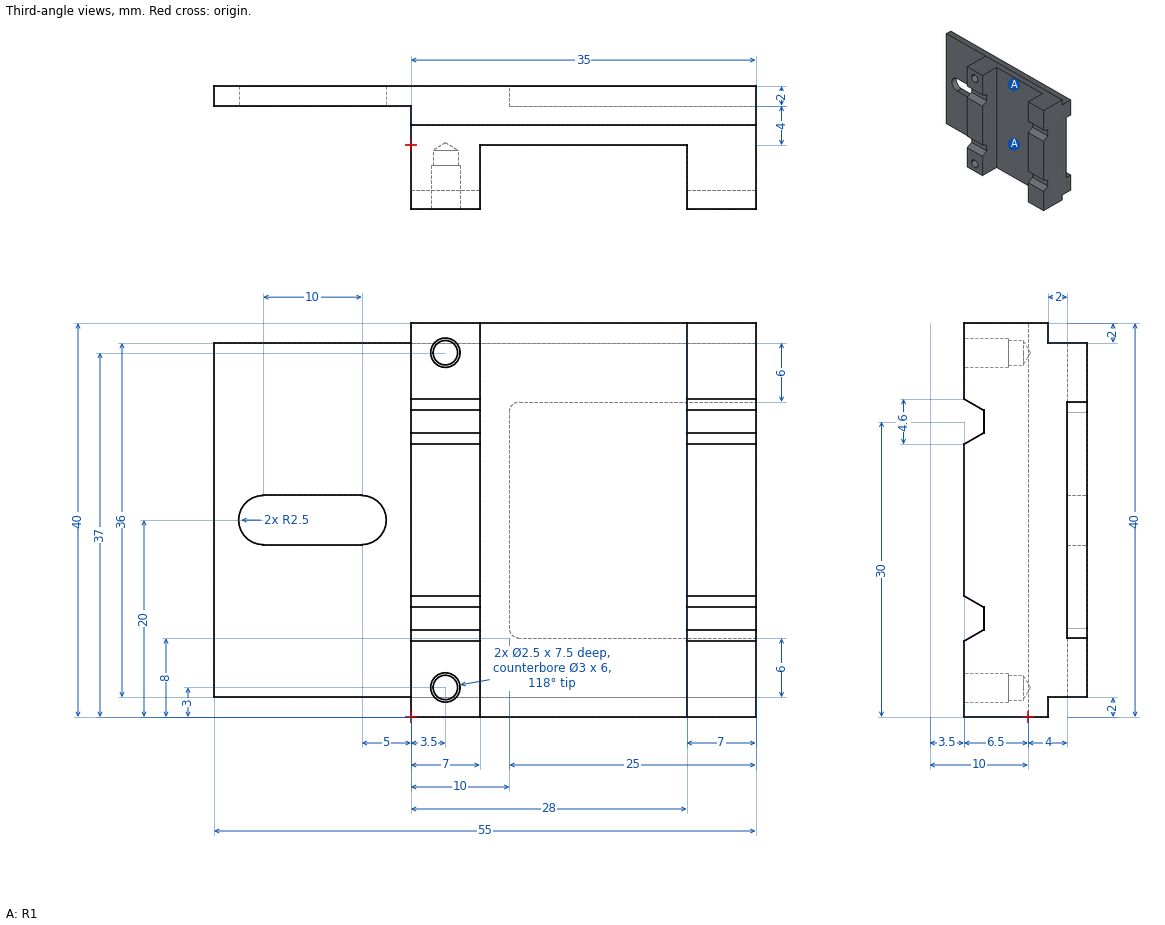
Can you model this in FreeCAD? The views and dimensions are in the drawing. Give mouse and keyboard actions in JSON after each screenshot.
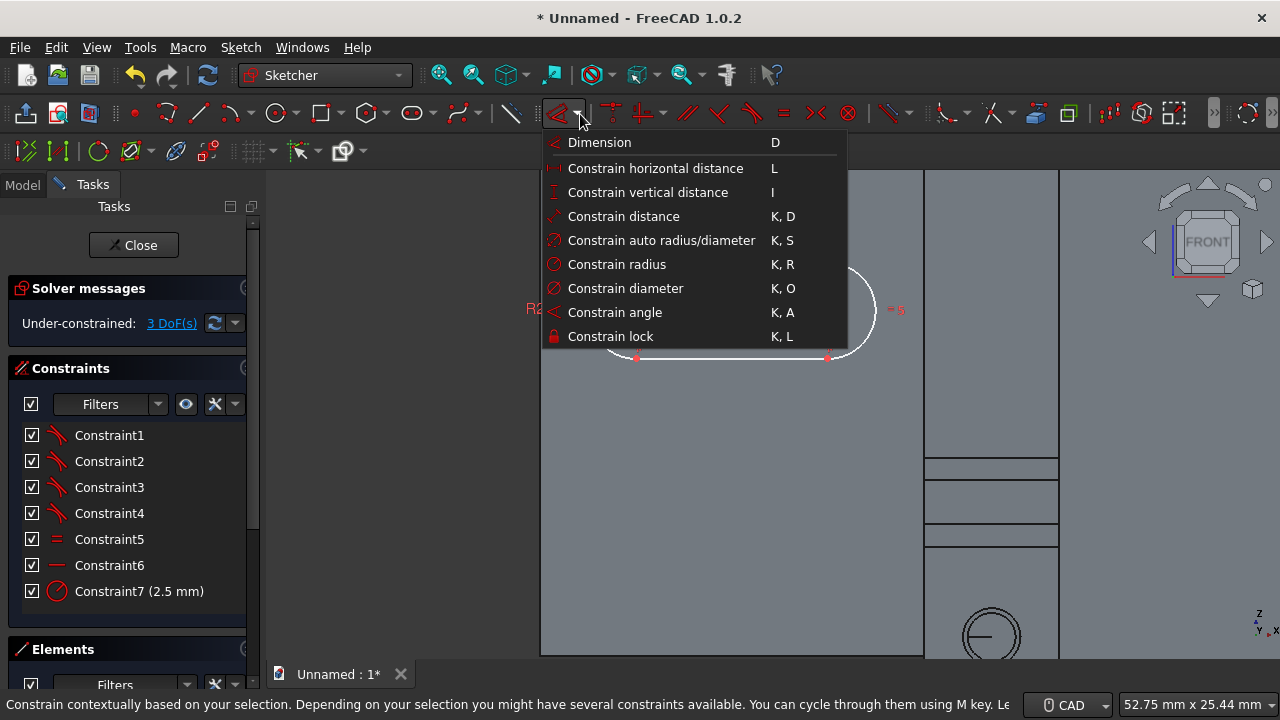
{"action": "left_click", "coordinate": [695, 168]}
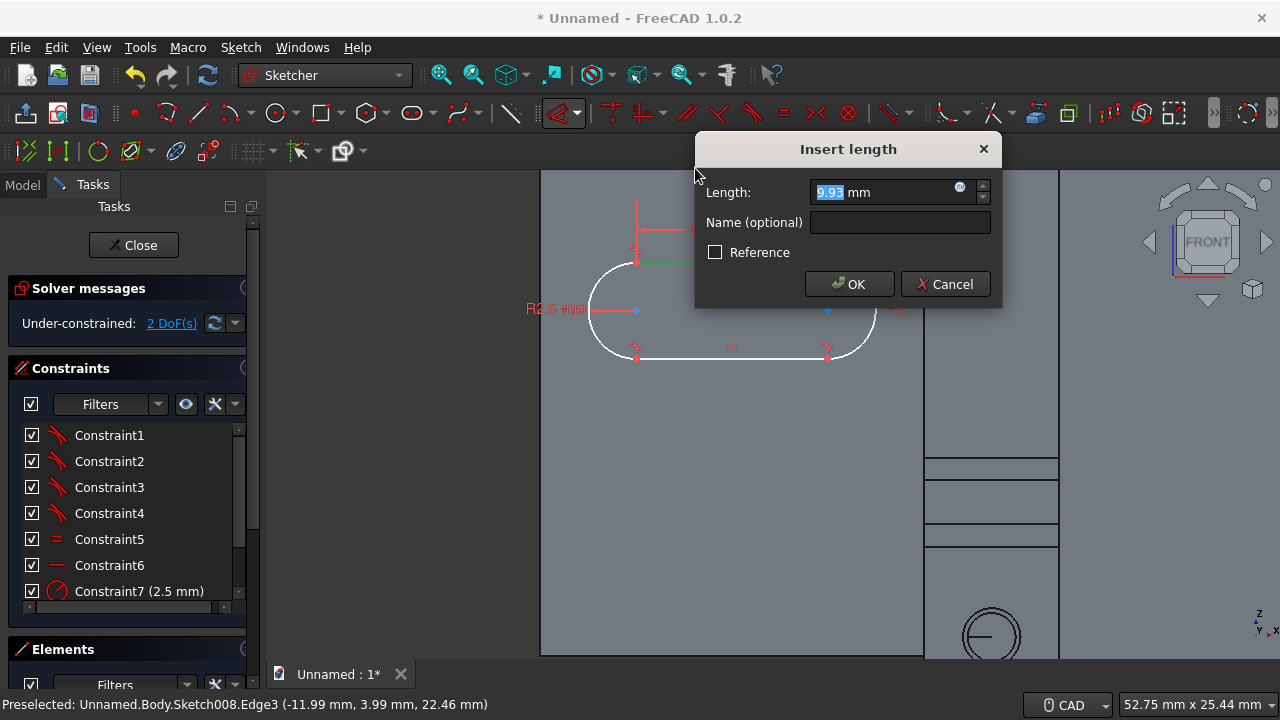
{"action": "type", "text": "10"}
{"action": "key", "text": "Return"}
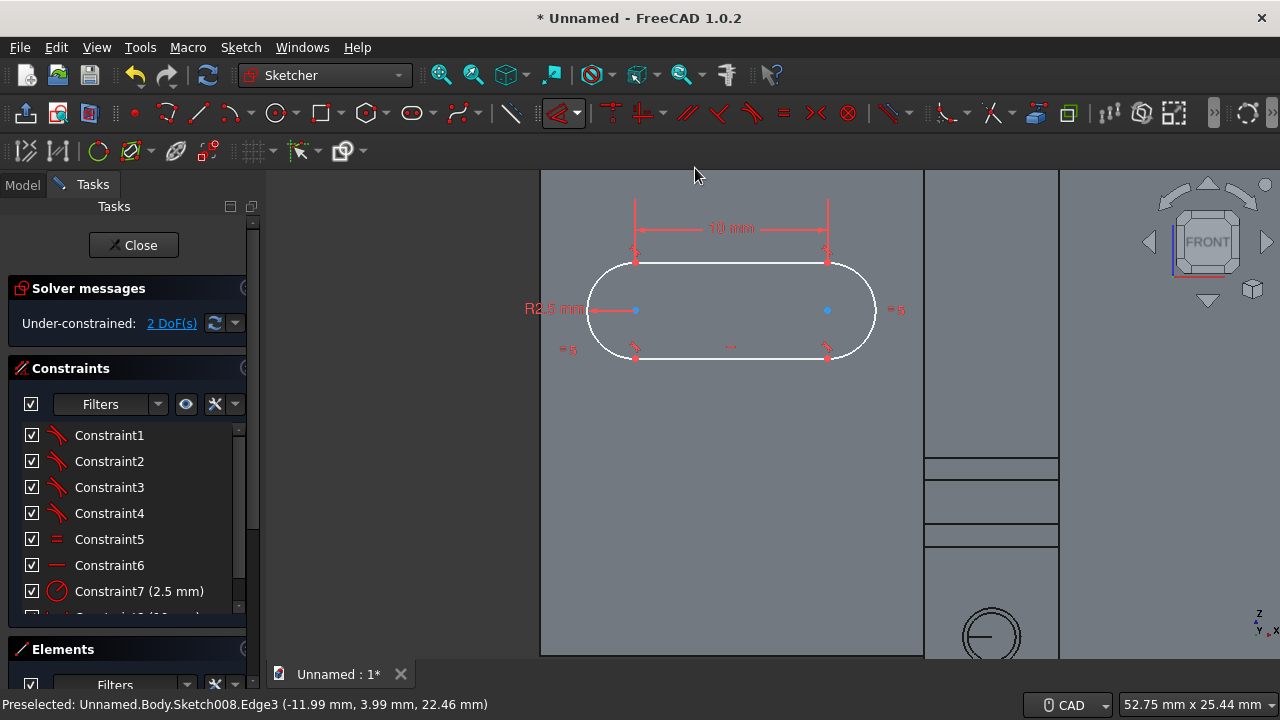
{"action": "left_click", "coordinate": [828, 359]}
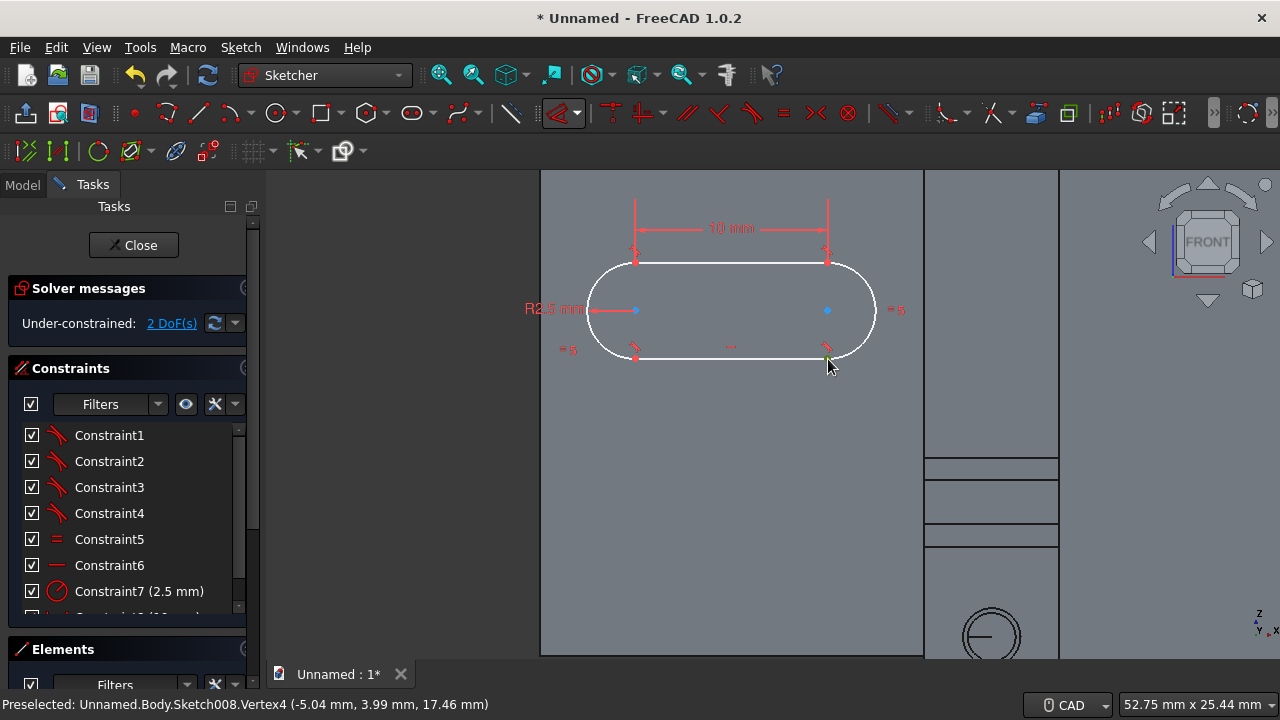
{"action": "key", "text": "l"}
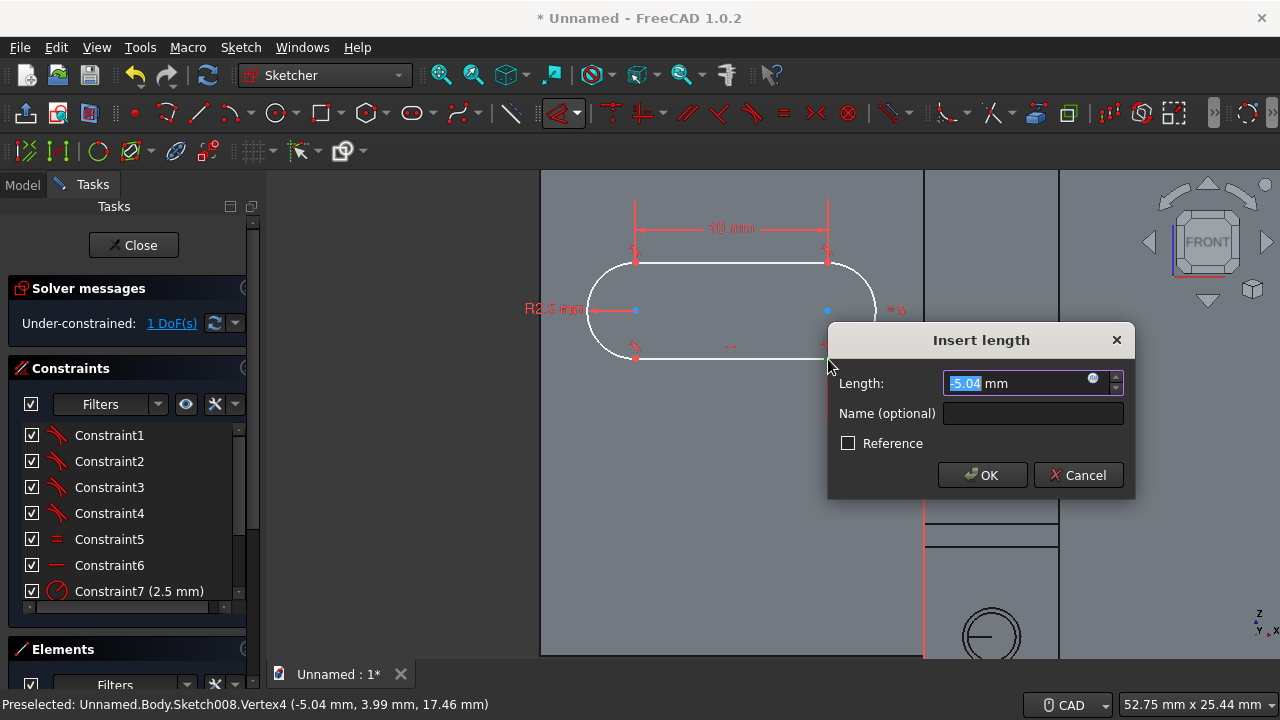
{"action": "type", "text": "-5"}
{"action": "key", "text": "Return"}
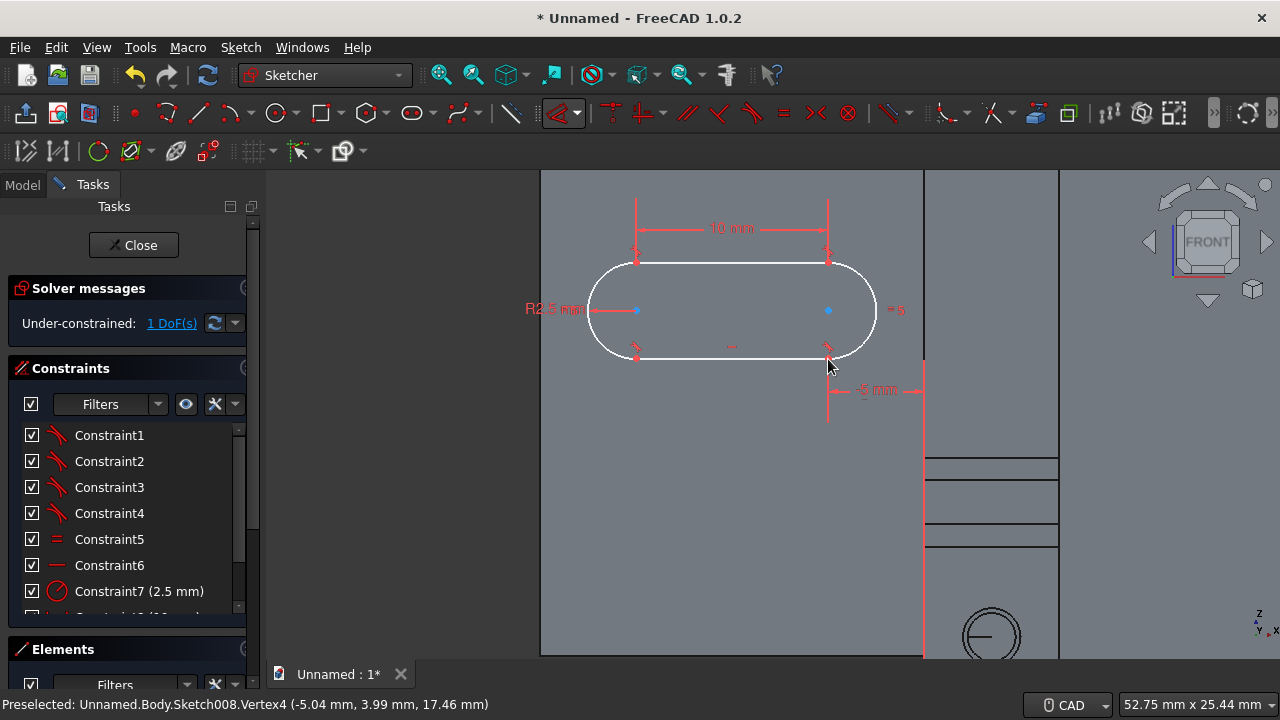
{"action": "left_click", "coordinate": [636, 311]}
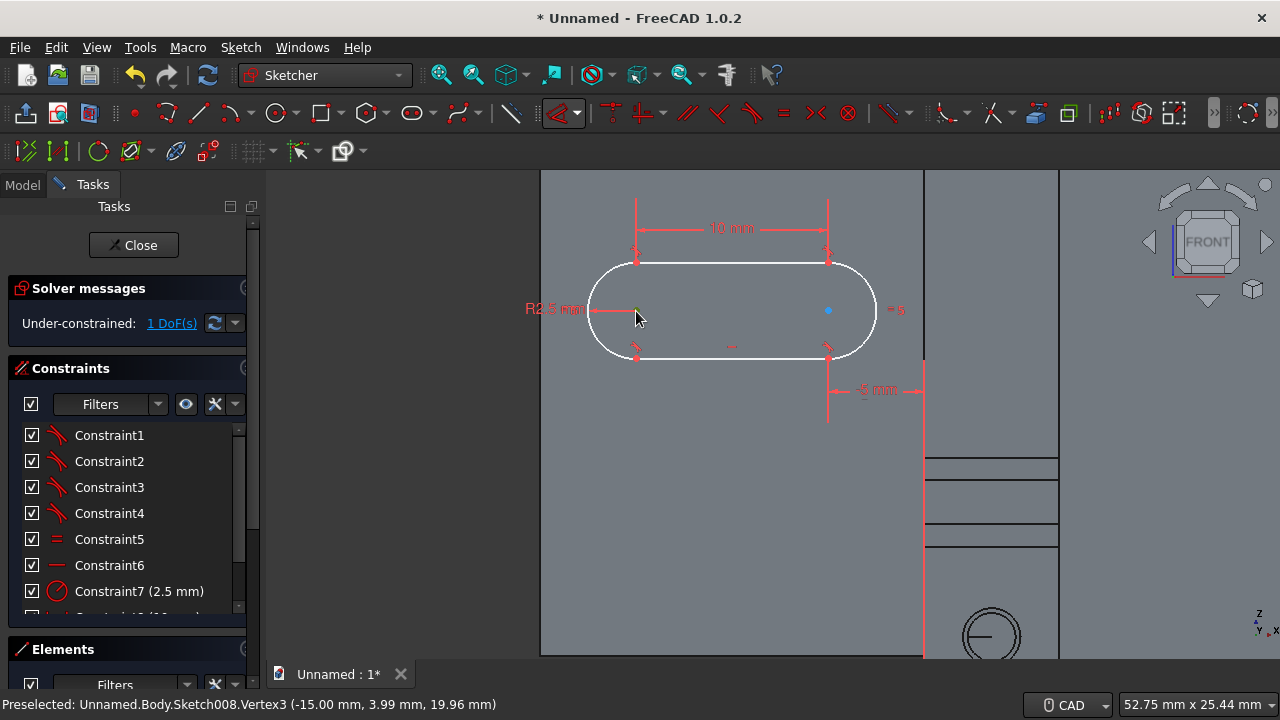
{"action": "left_click", "coordinate": [580, 114]}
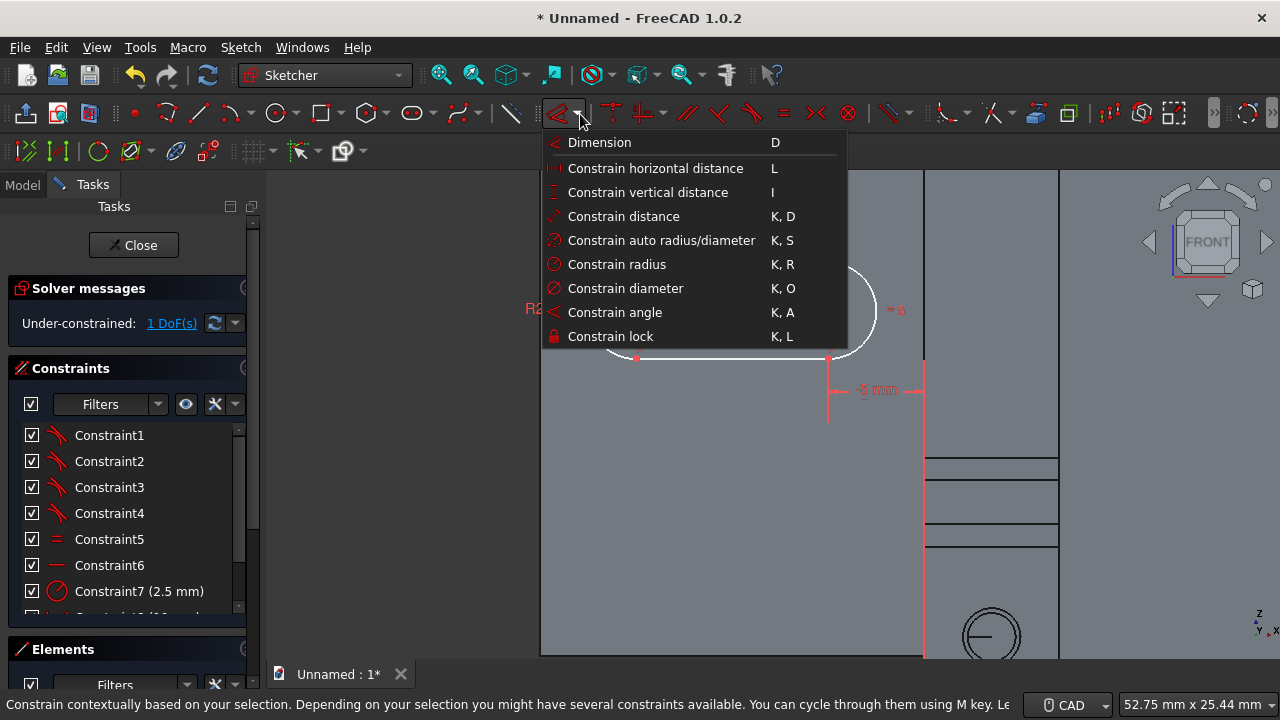
{"action": "left_click", "coordinate": [695, 192]}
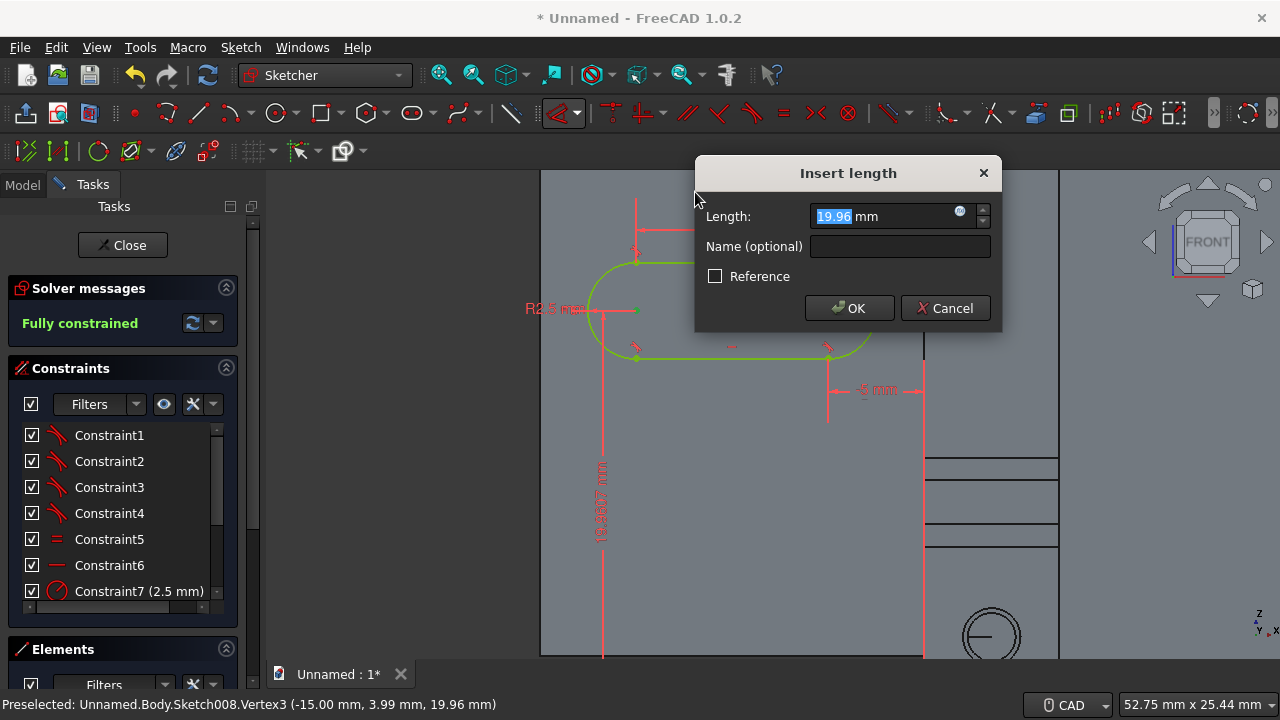
{"action": "type", "text": "20"}
{"action": "key", "text": "Return"}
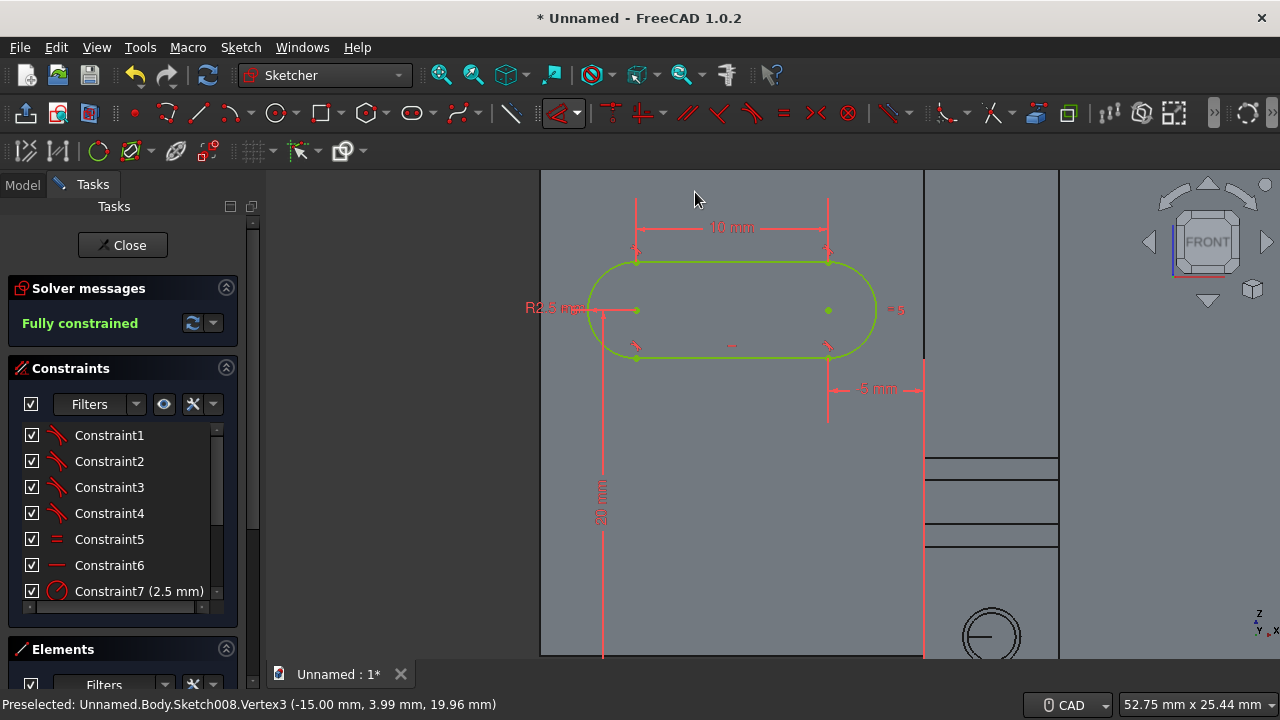
{"action": "left_click", "coordinate": [123, 245]}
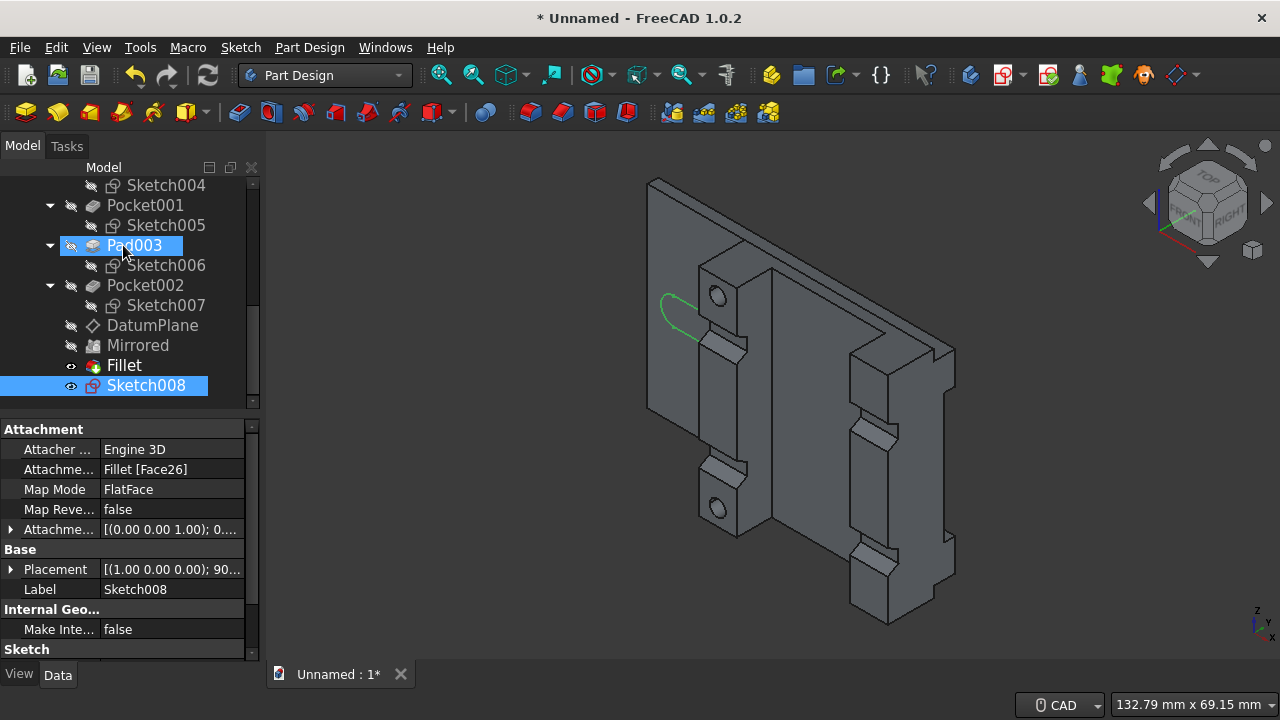
{"action": "left_click", "coordinate": [240, 112]}